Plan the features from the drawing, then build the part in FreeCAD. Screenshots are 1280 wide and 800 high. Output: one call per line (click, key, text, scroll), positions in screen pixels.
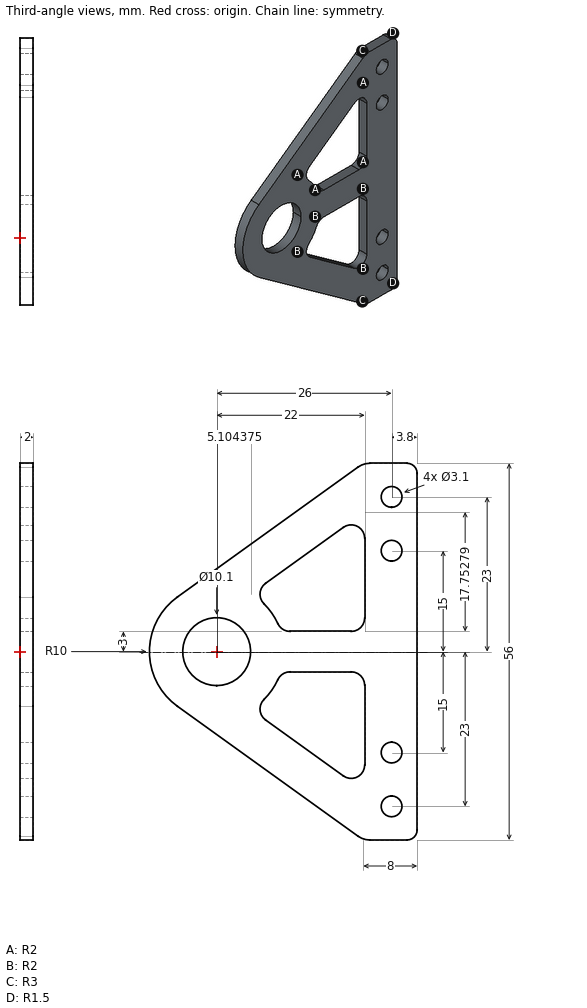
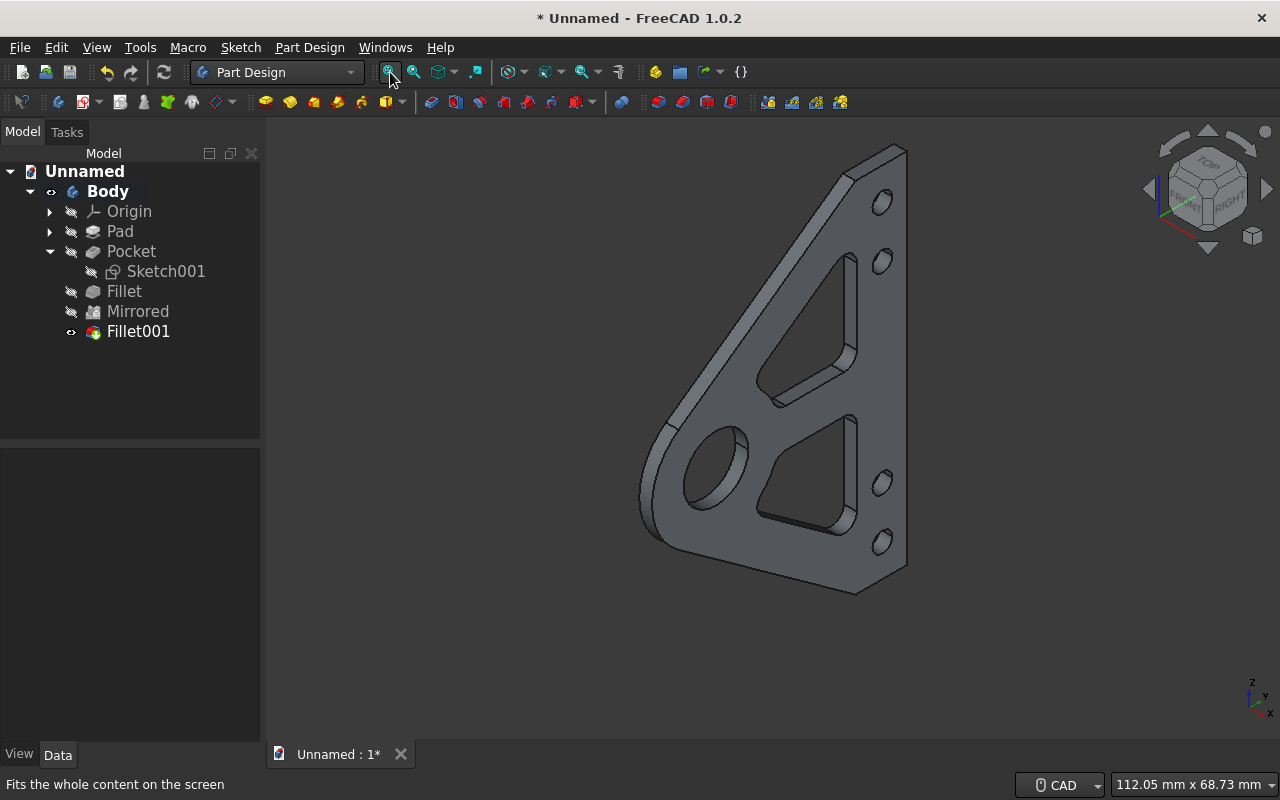
key(2)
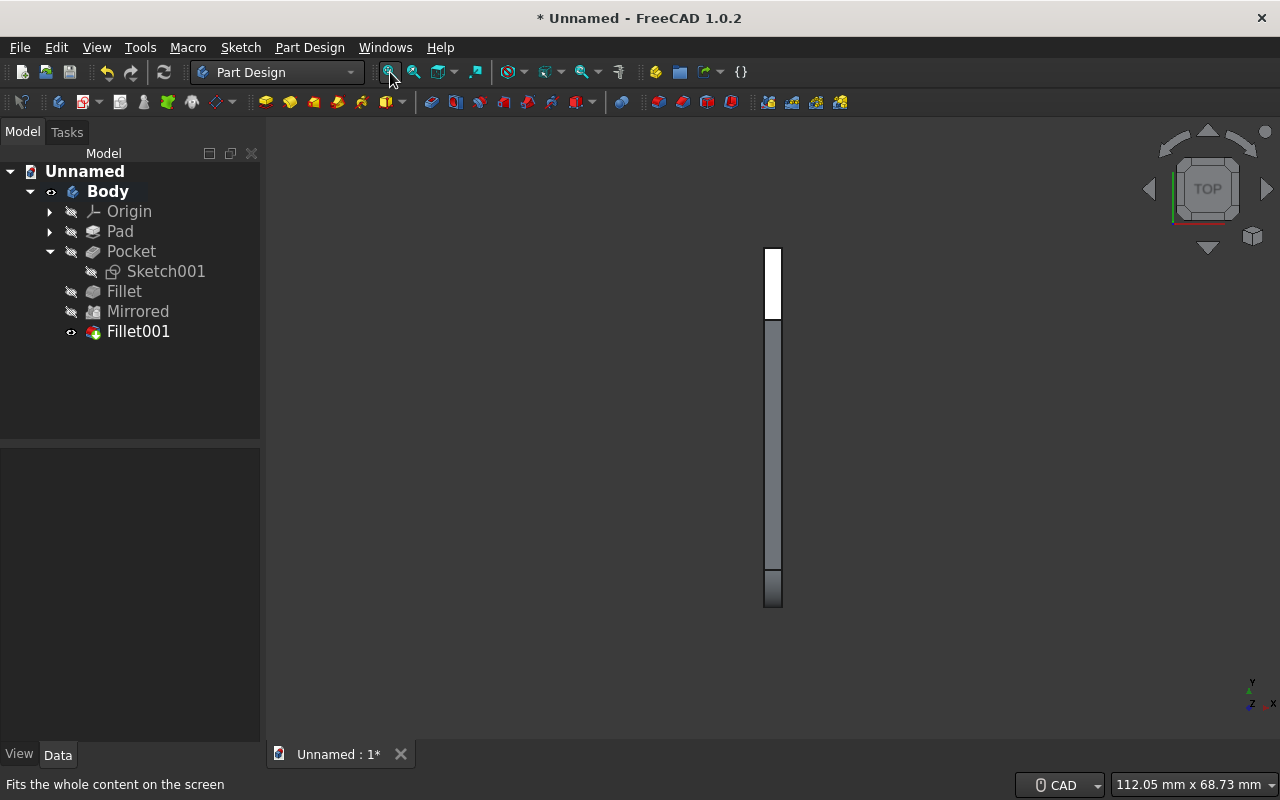
click(773, 319)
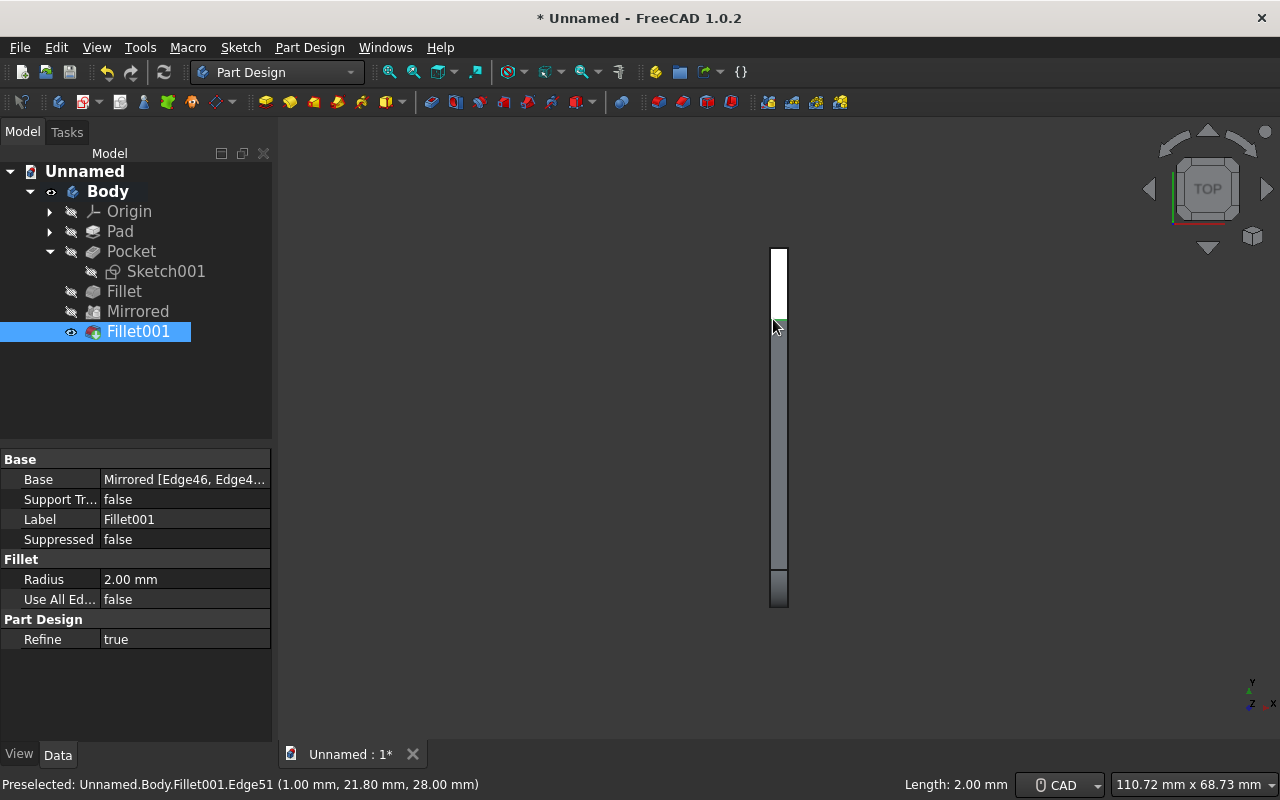
scroll(779, 319, up, 4)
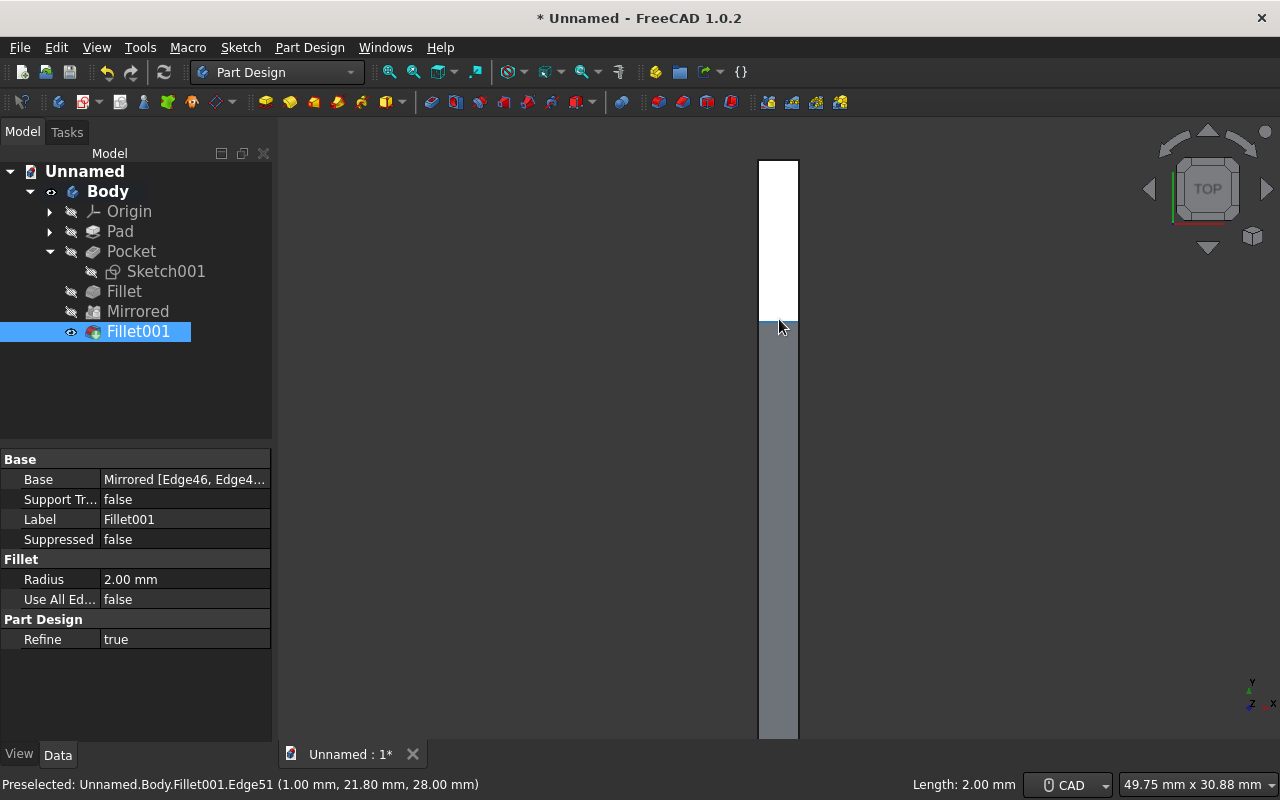
key(v)
key(f)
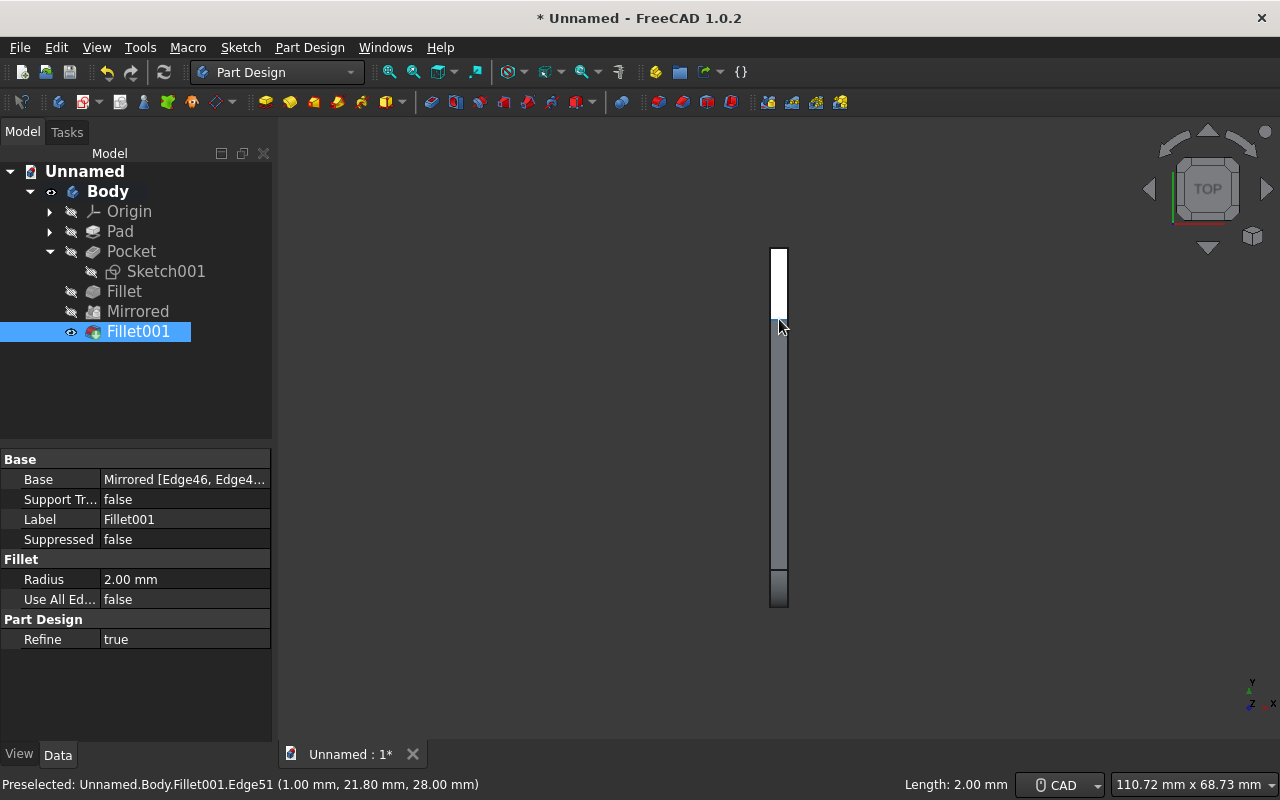
key(0)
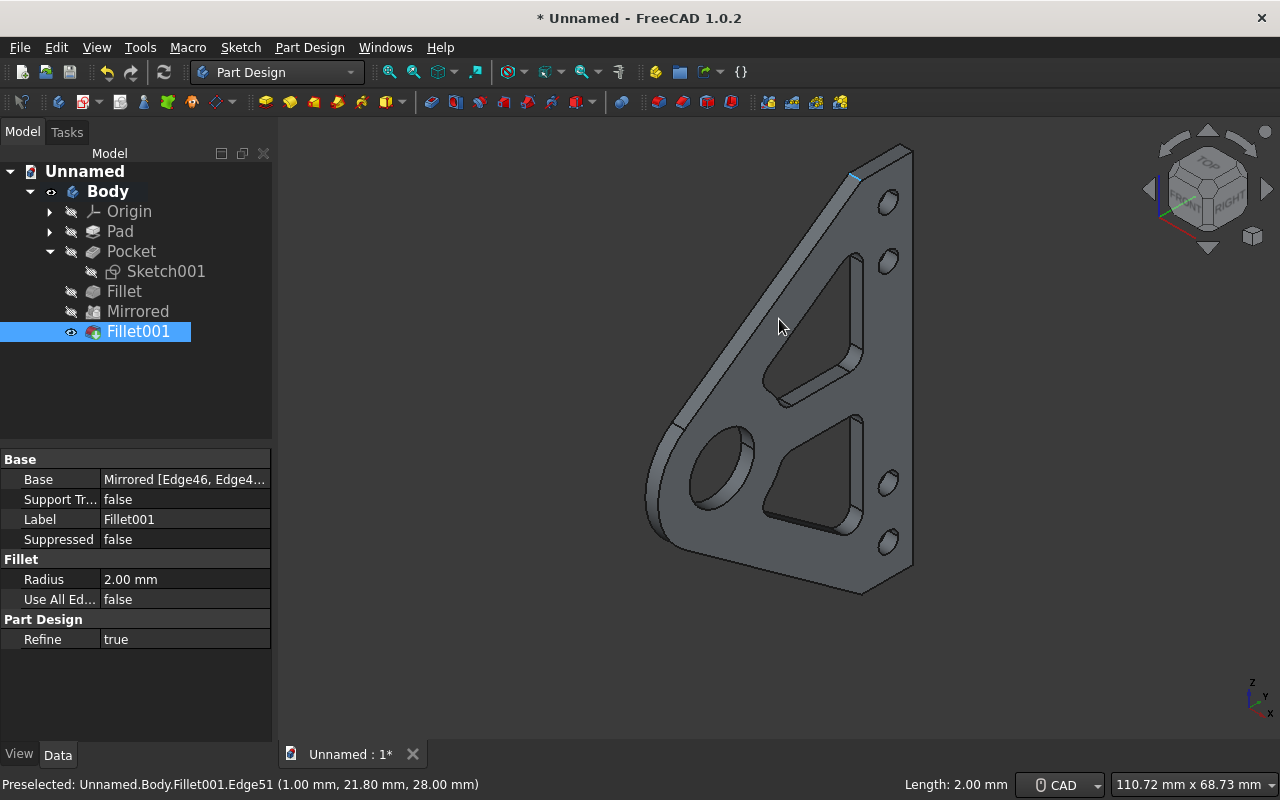
scroll(855, 590, up, 4)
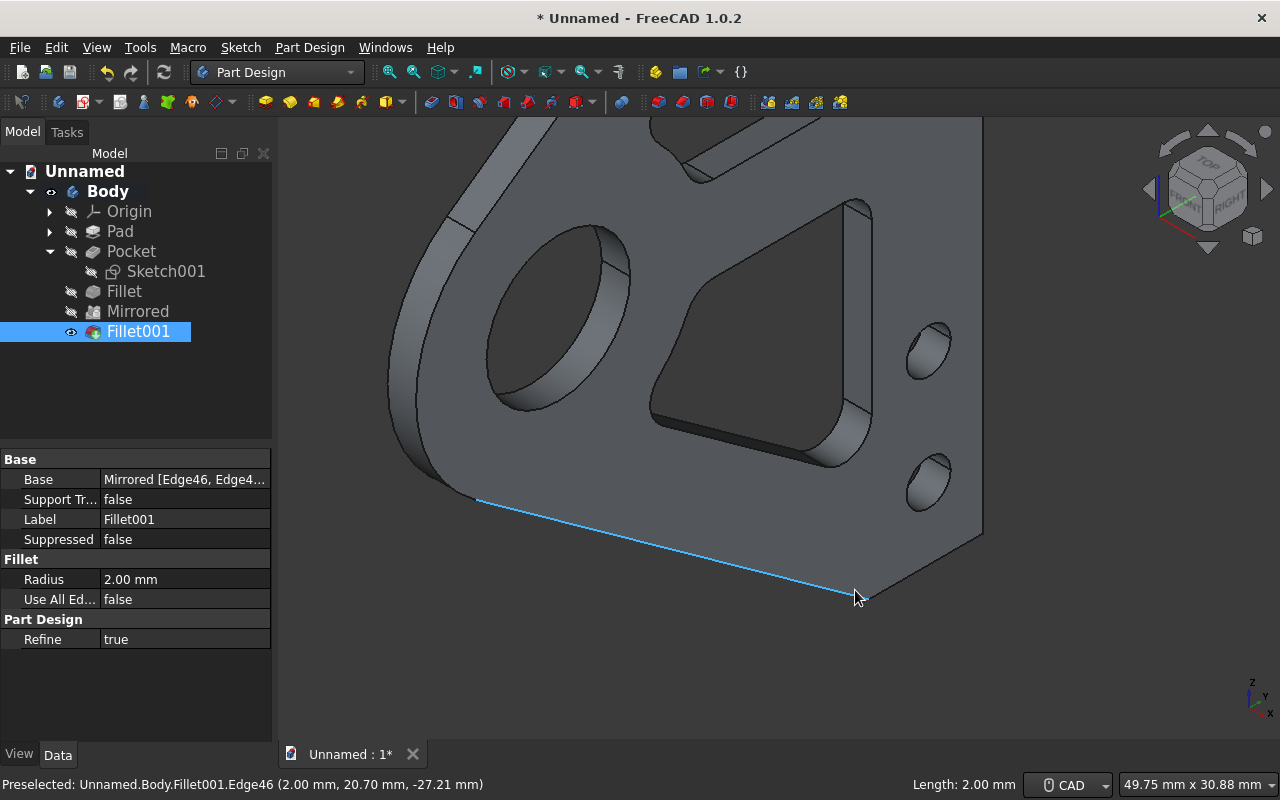
click(390, 72)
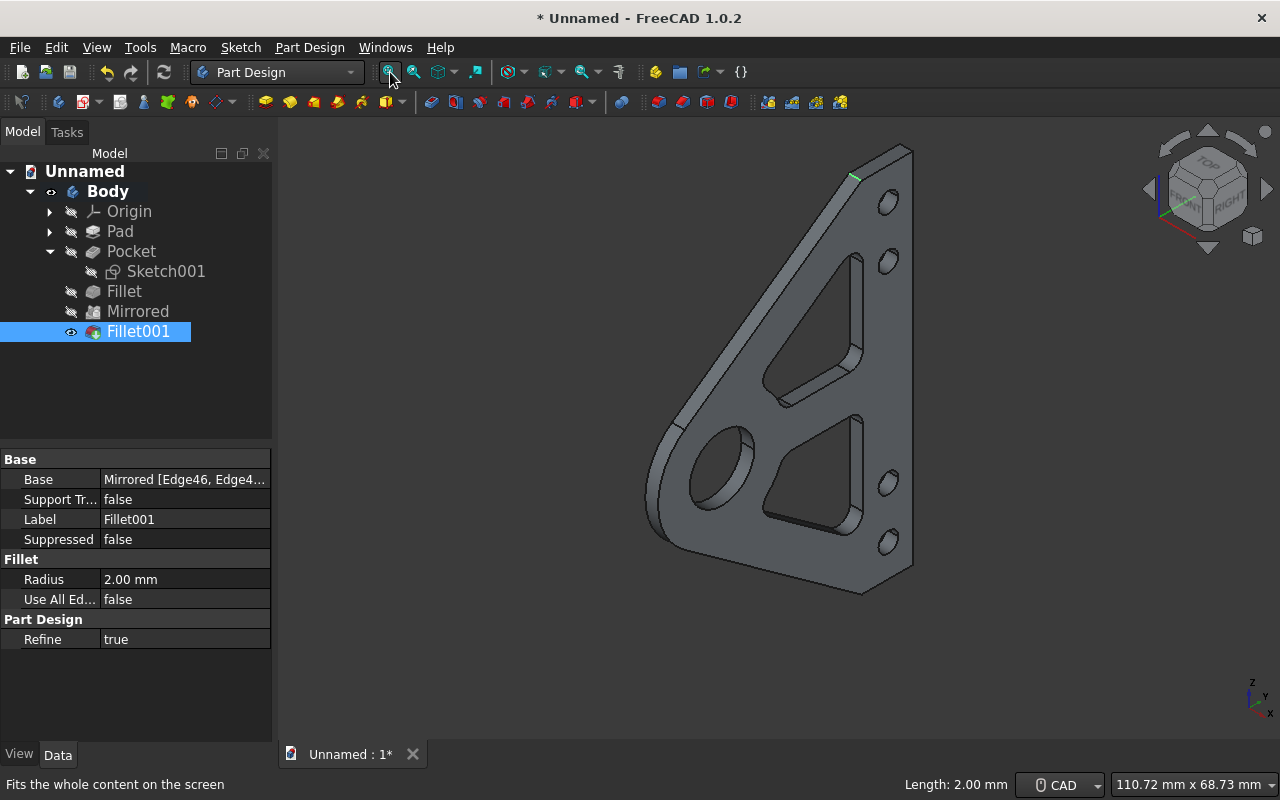
key(1)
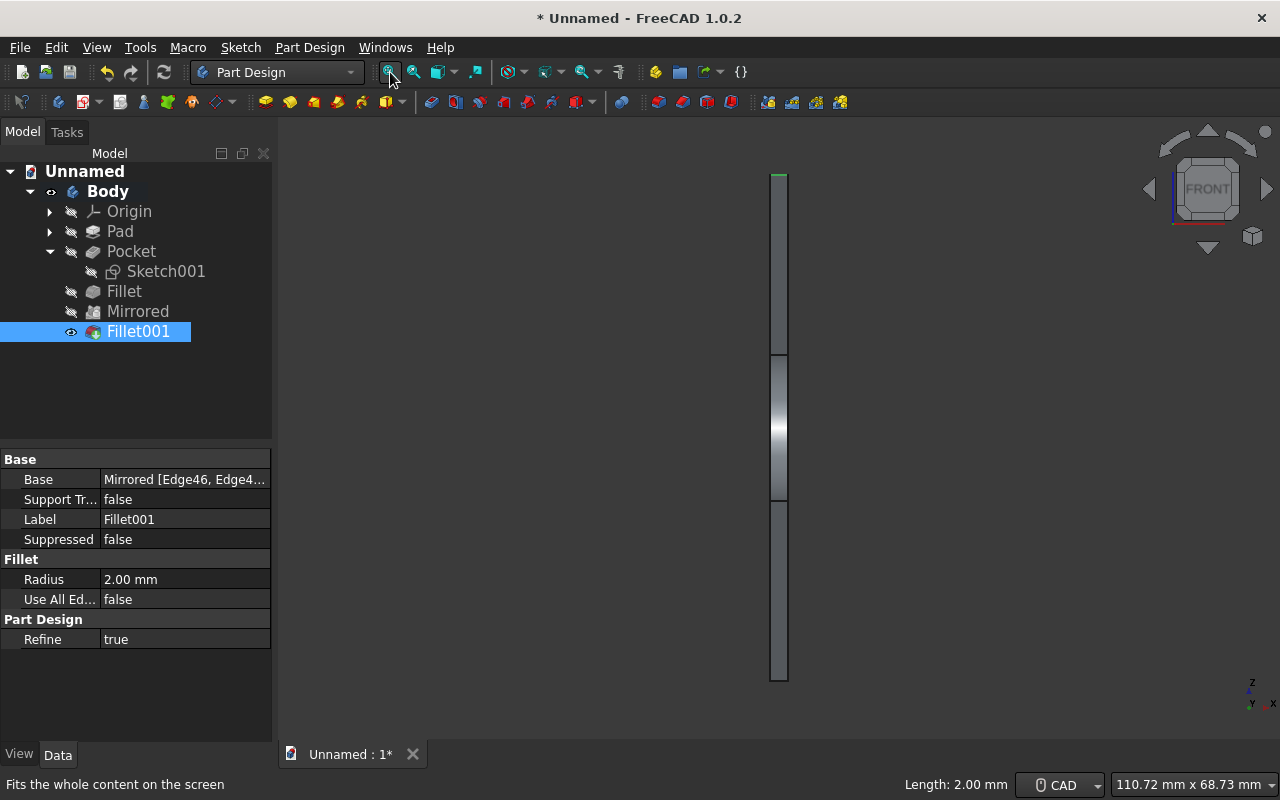
scroll(779, 680, up, 4)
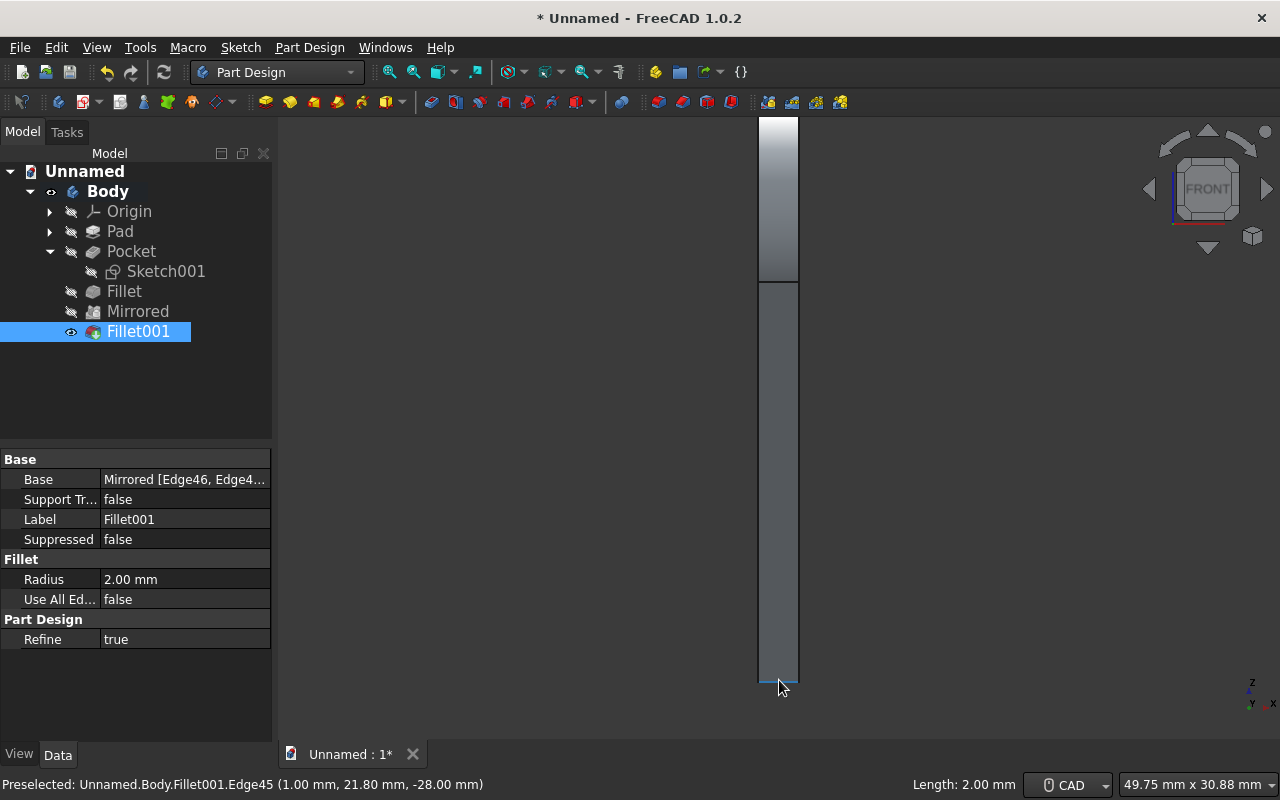
click(390, 72)